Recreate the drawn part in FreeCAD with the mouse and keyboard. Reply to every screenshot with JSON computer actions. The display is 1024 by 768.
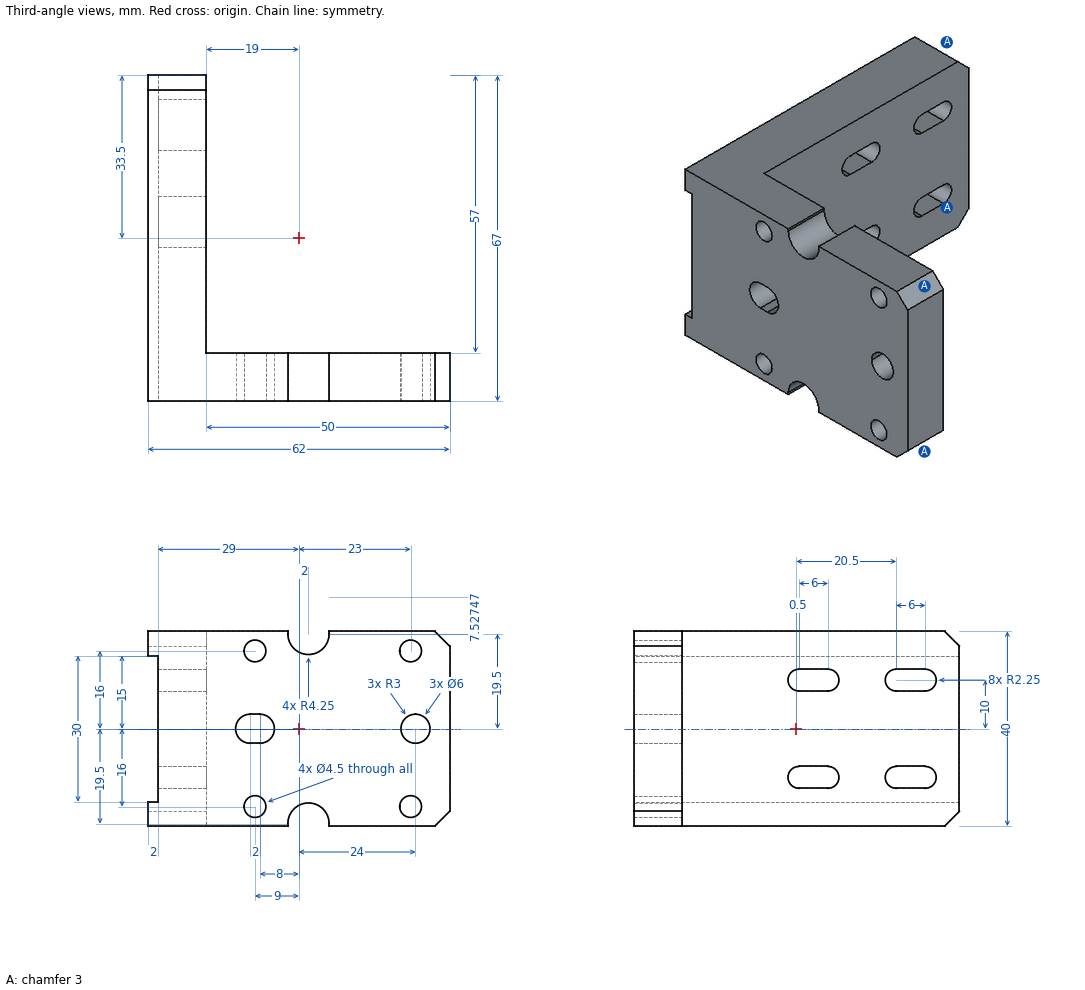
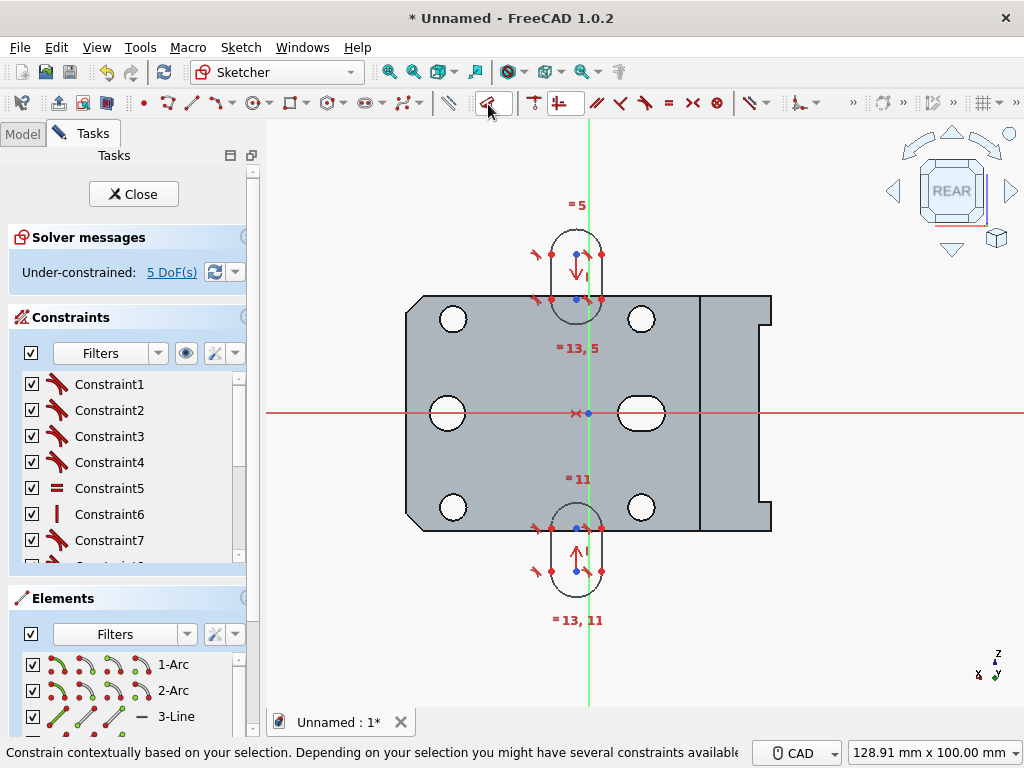
{"action": "scroll", "coordinate": [562, 320], "scroll_direction": "up", "scroll_amount": 3}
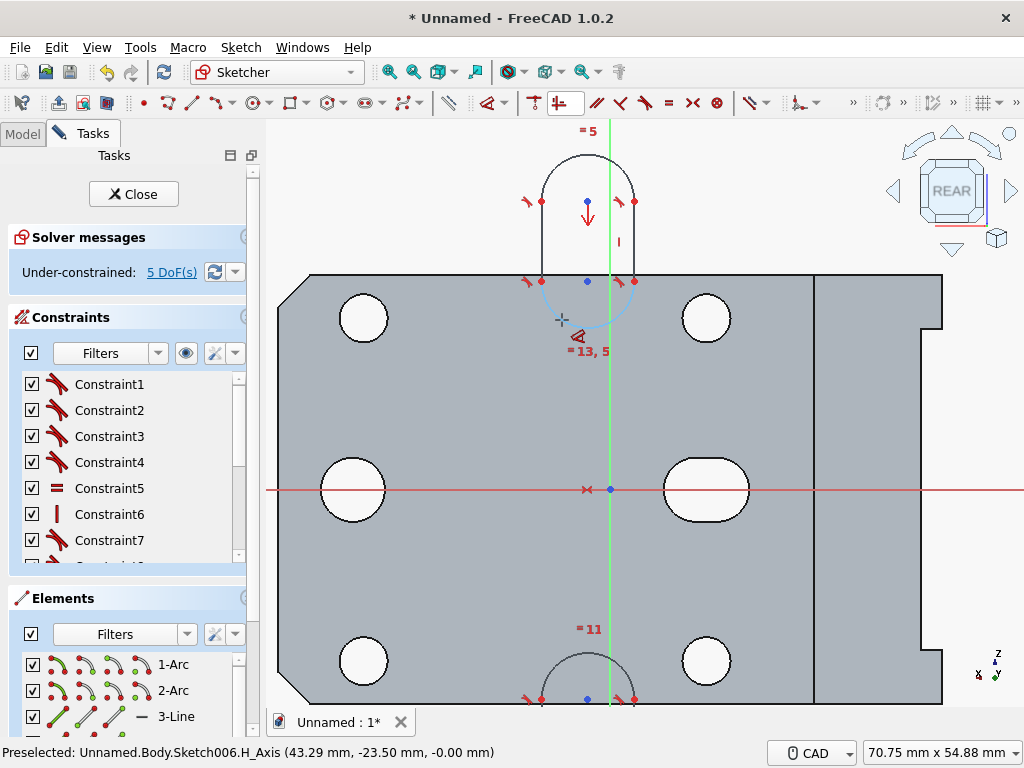
{"action": "left_click", "coordinate": [561, 319]}
{"action": "left_click", "coordinate": [542, 345]}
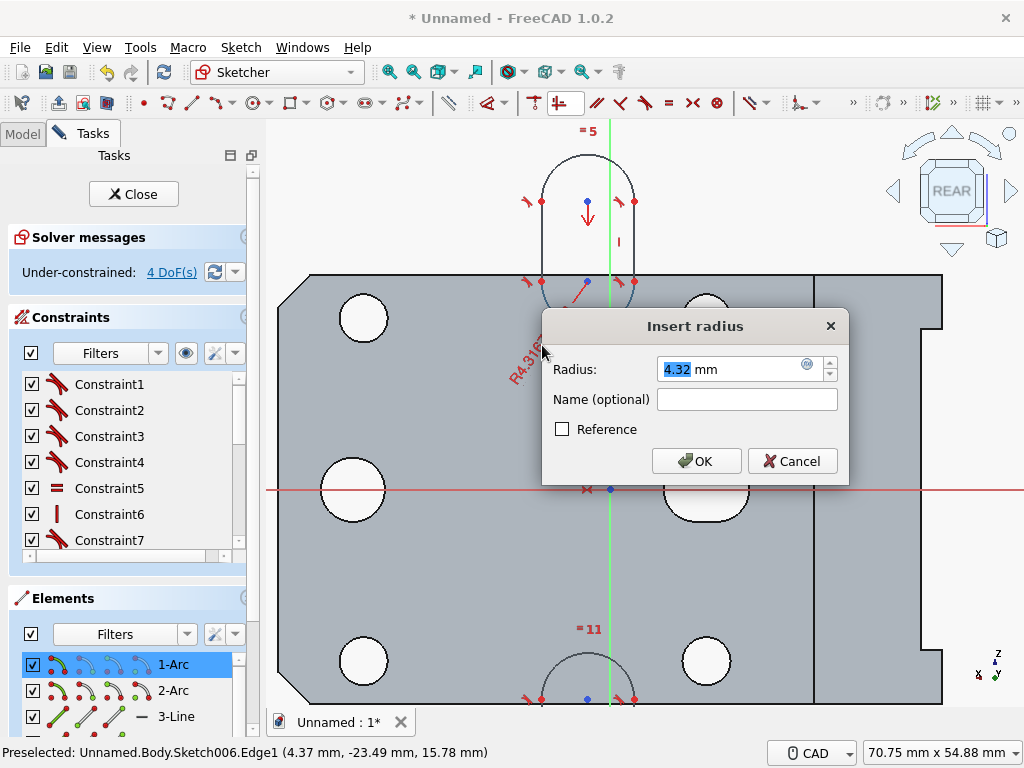
{"action": "type", "text": "4.25"}
{"action": "key", "text": "Return"}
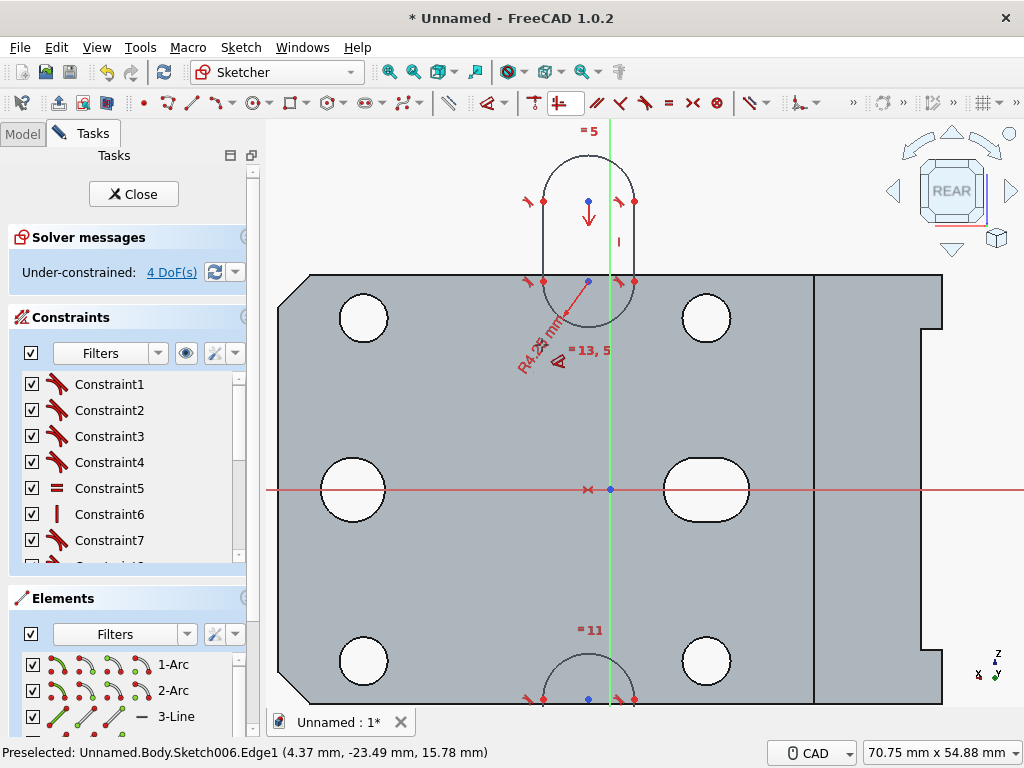
{"action": "scroll", "coordinate": [589, 282], "scroll_direction": "up", "scroll_amount": 4}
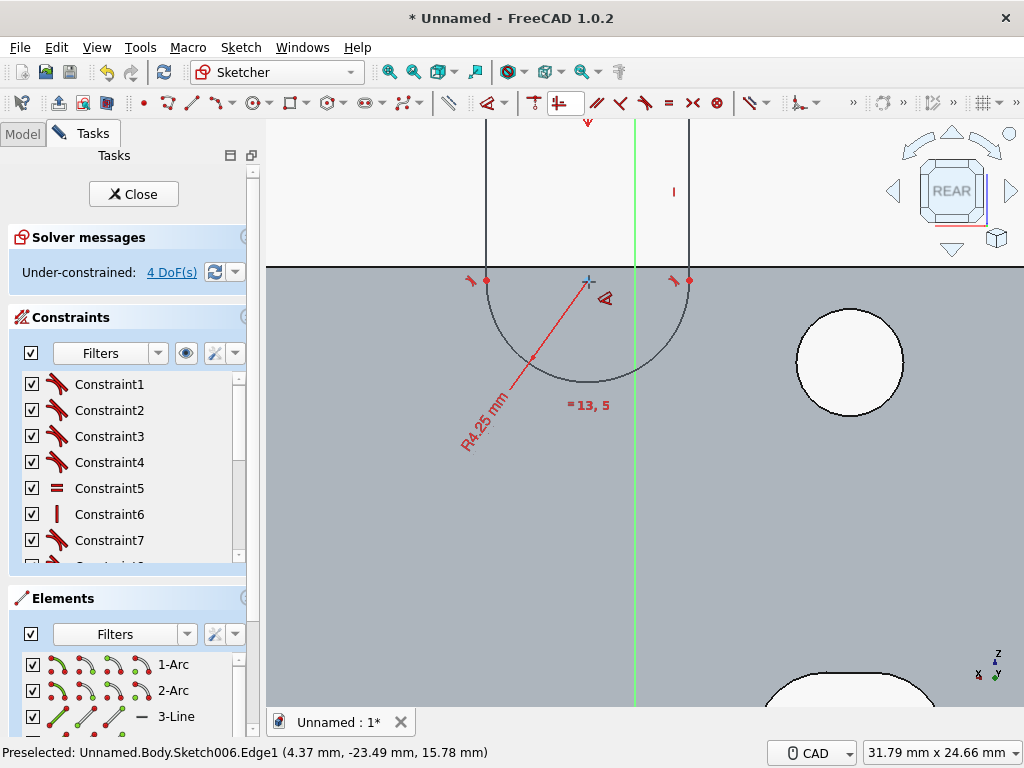
{"action": "left_click", "coordinate": [588, 281]}
{"action": "left_click", "coordinate": [612, 247]}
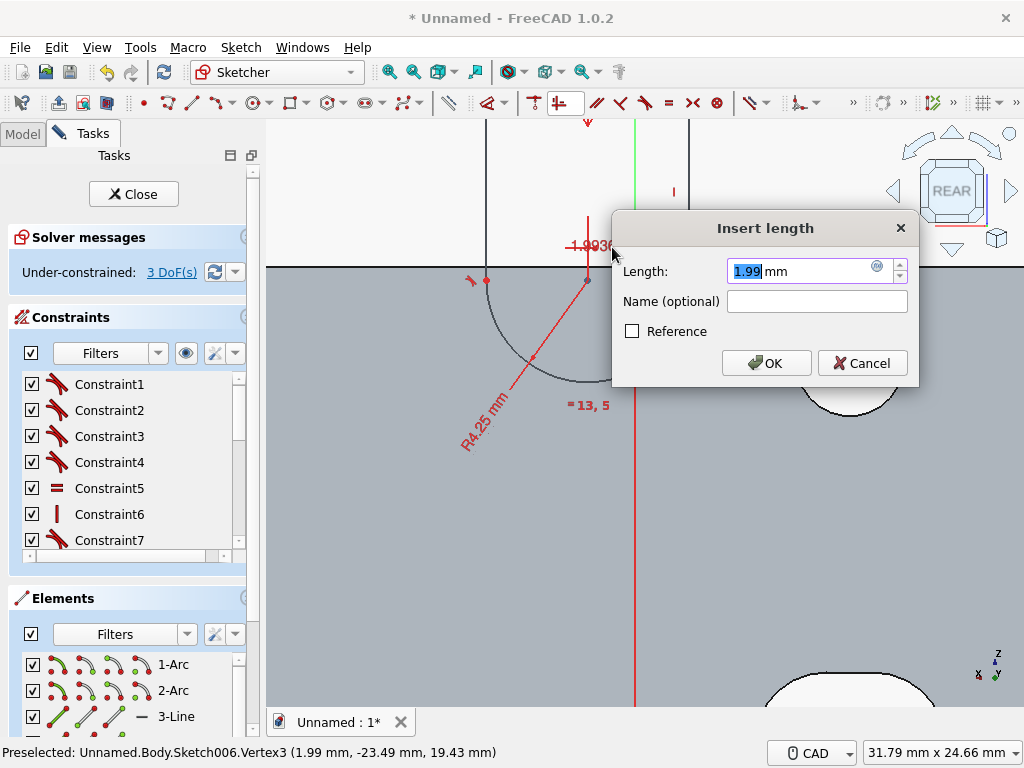
{"action": "type", "text": "2"}
{"action": "key", "text": "Return"}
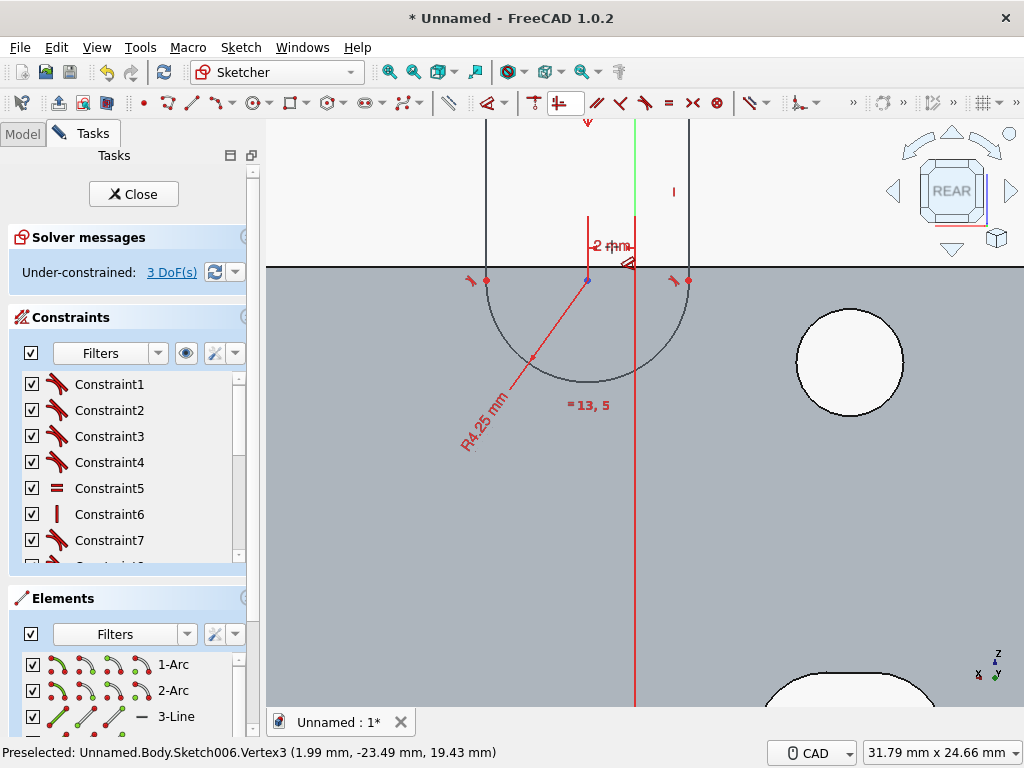
{"action": "scroll", "coordinate": [573, 305], "scroll_direction": "down", "scroll_amount": 7}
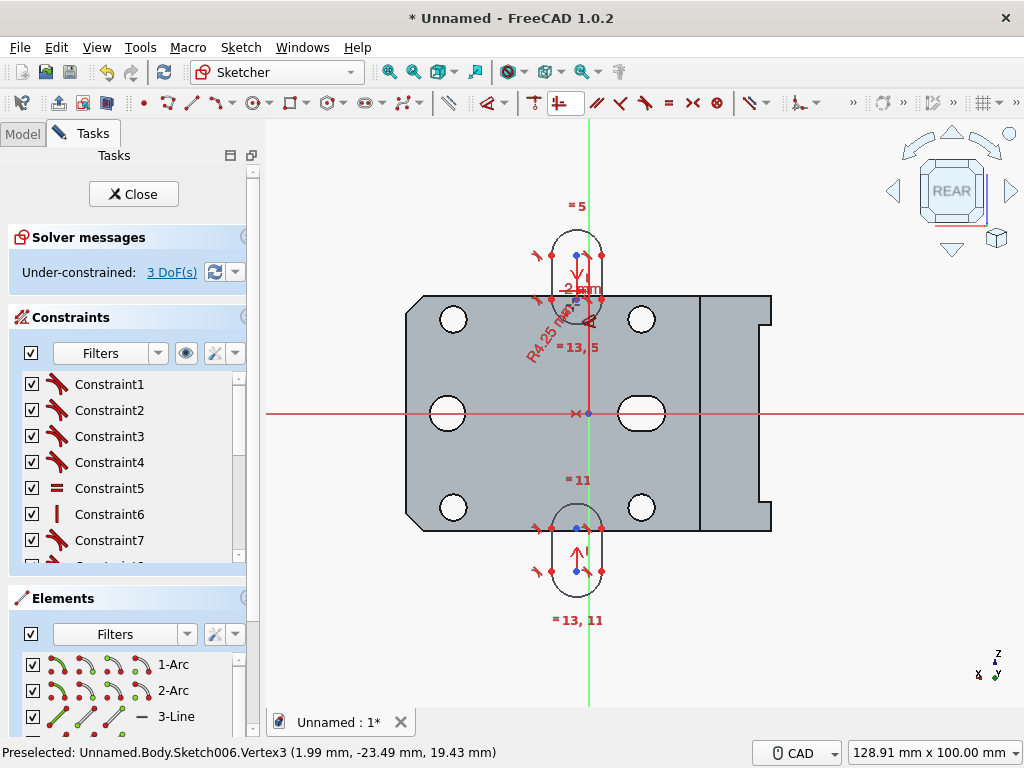
{"action": "left_click", "coordinate": [552, 299]}
{"action": "left_click", "coordinate": [518, 356]}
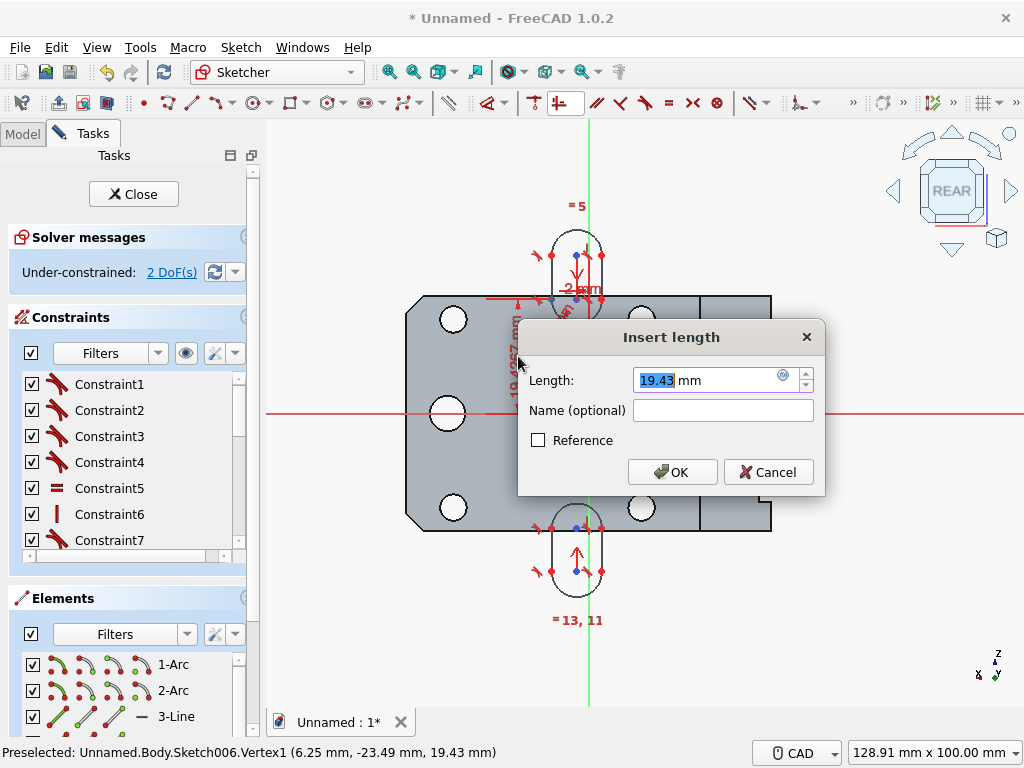
{"action": "type", "text": "19.5"}
{"action": "key", "text": "Return"}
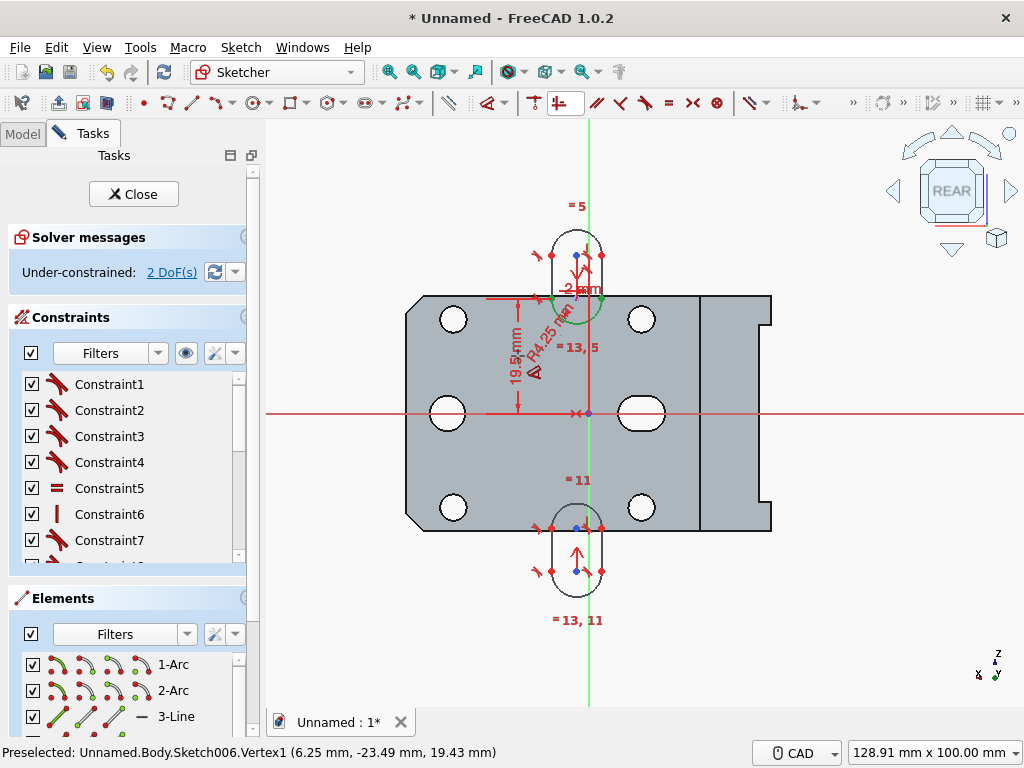
{"action": "left_click", "coordinate": [602, 529]}
{"action": "left_click", "coordinate": [636, 471]}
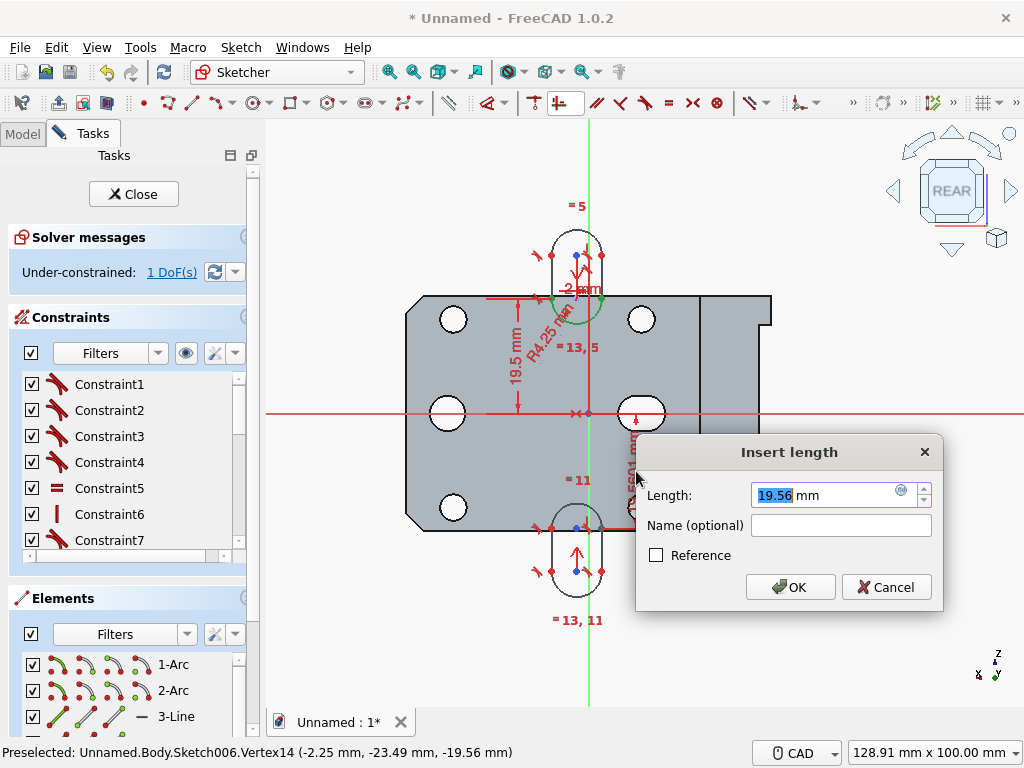
{"action": "type", "text": "19.5"}
{"action": "key", "text": "Return"}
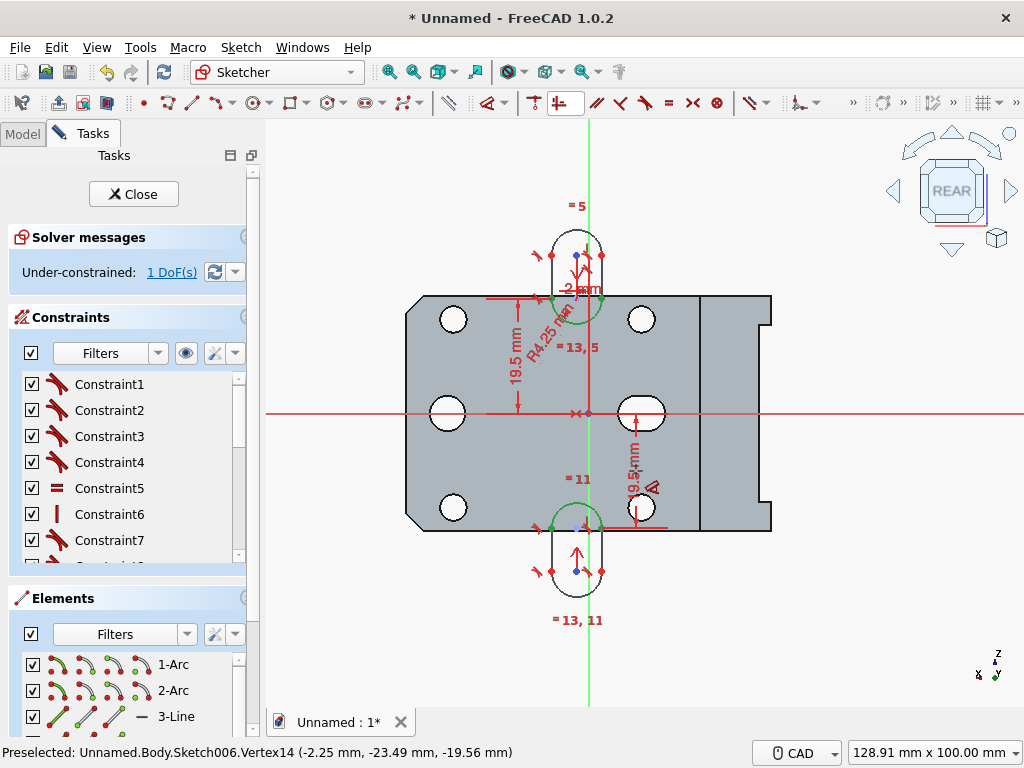
{"action": "left_click", "coordinate": [552, 286]}
{"action": "left_click", "coordinate": [518, 267]}